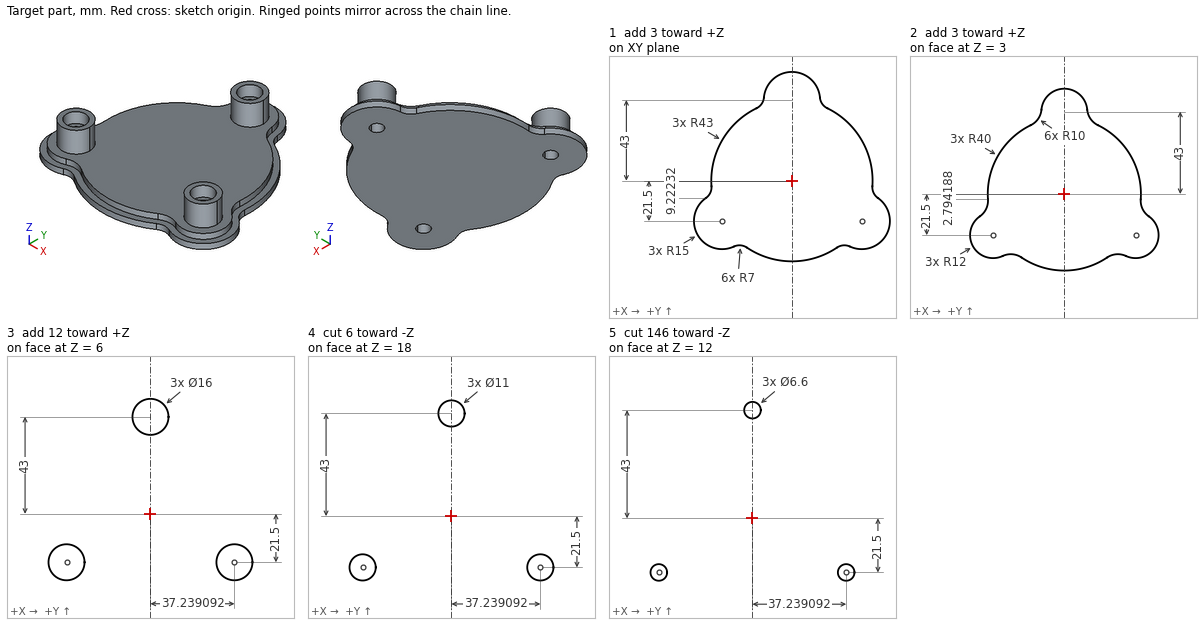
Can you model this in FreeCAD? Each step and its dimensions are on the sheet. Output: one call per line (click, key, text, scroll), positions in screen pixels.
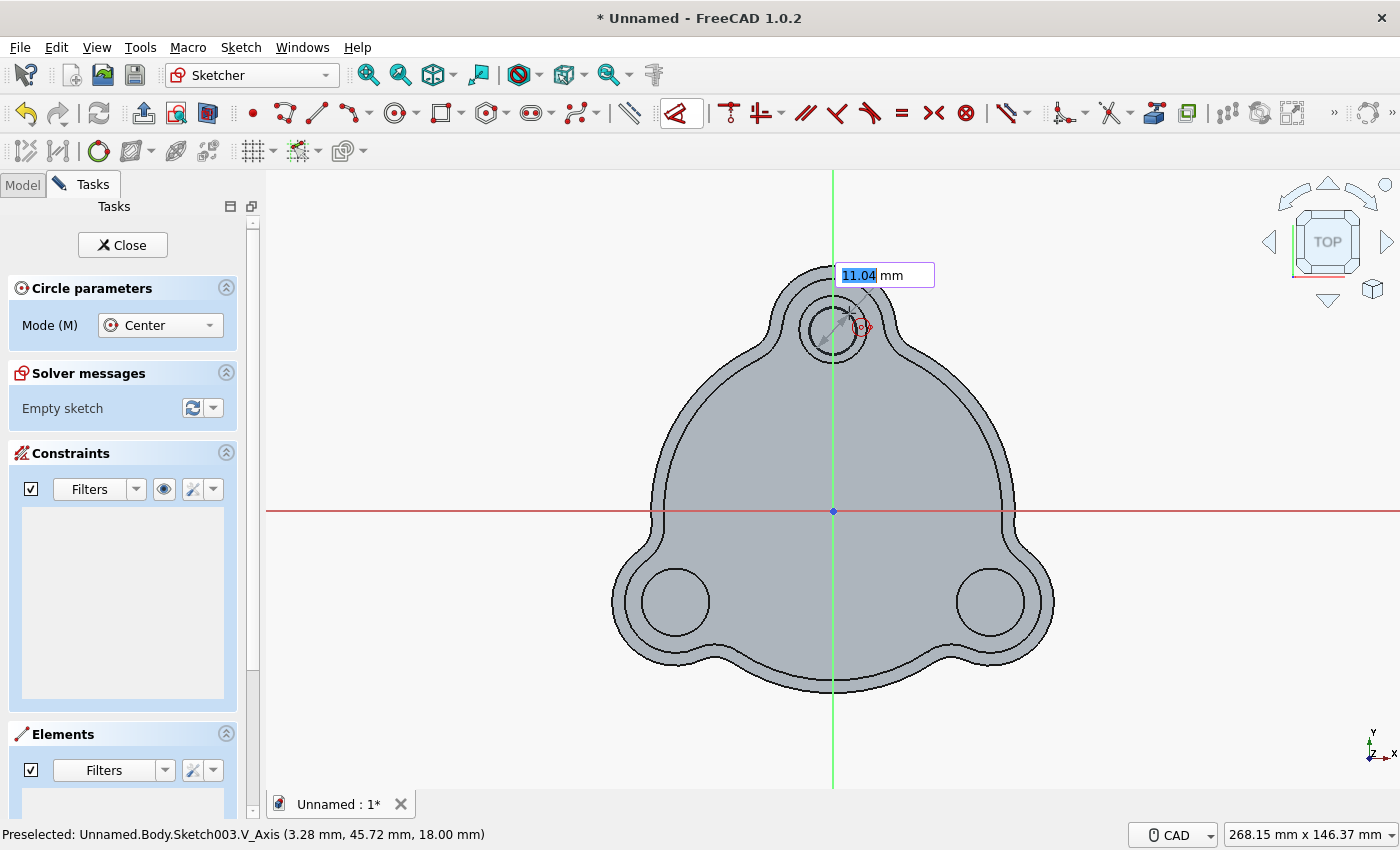
text(11)
key(Return)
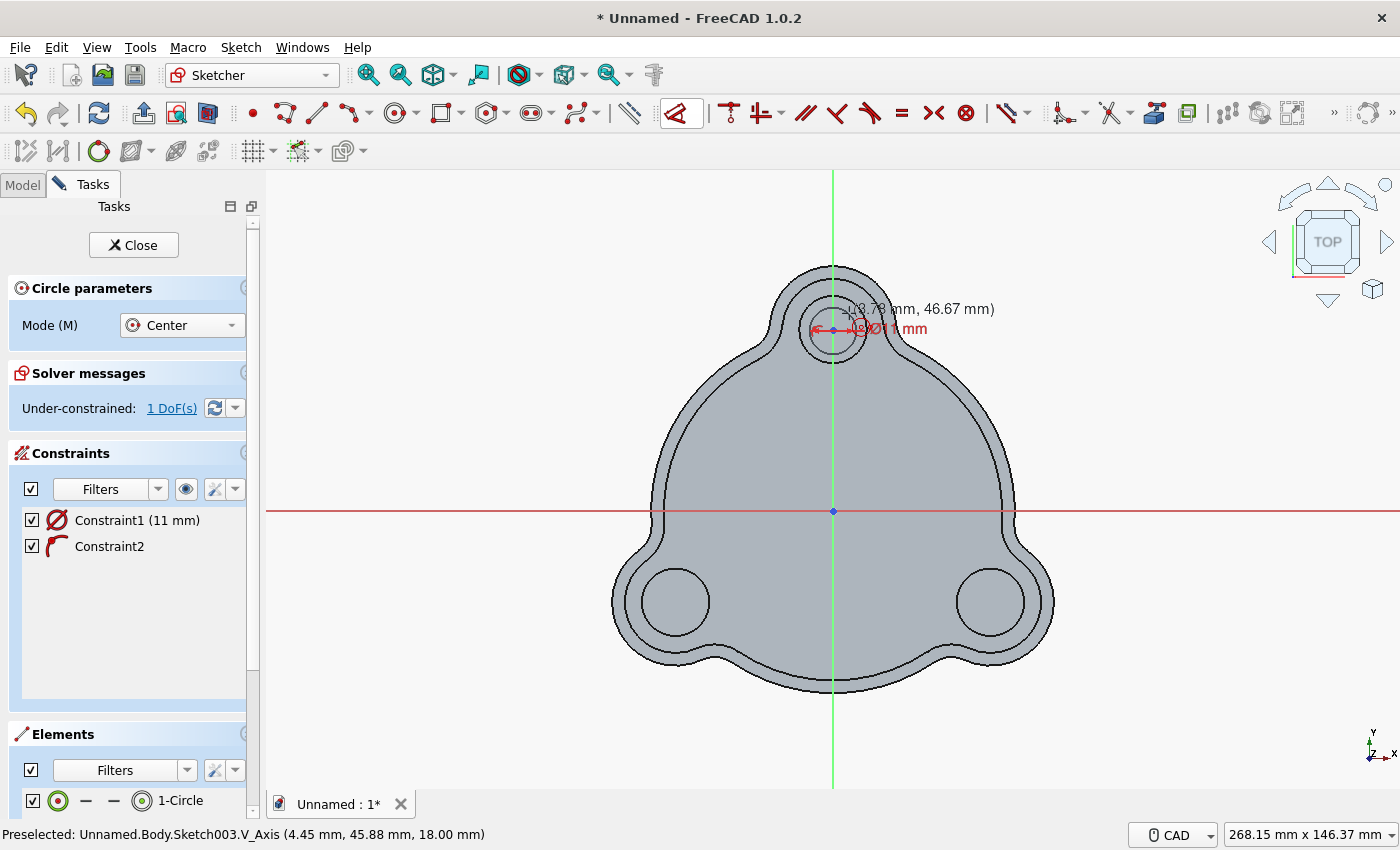
click(990, 602)
move(1007, 586)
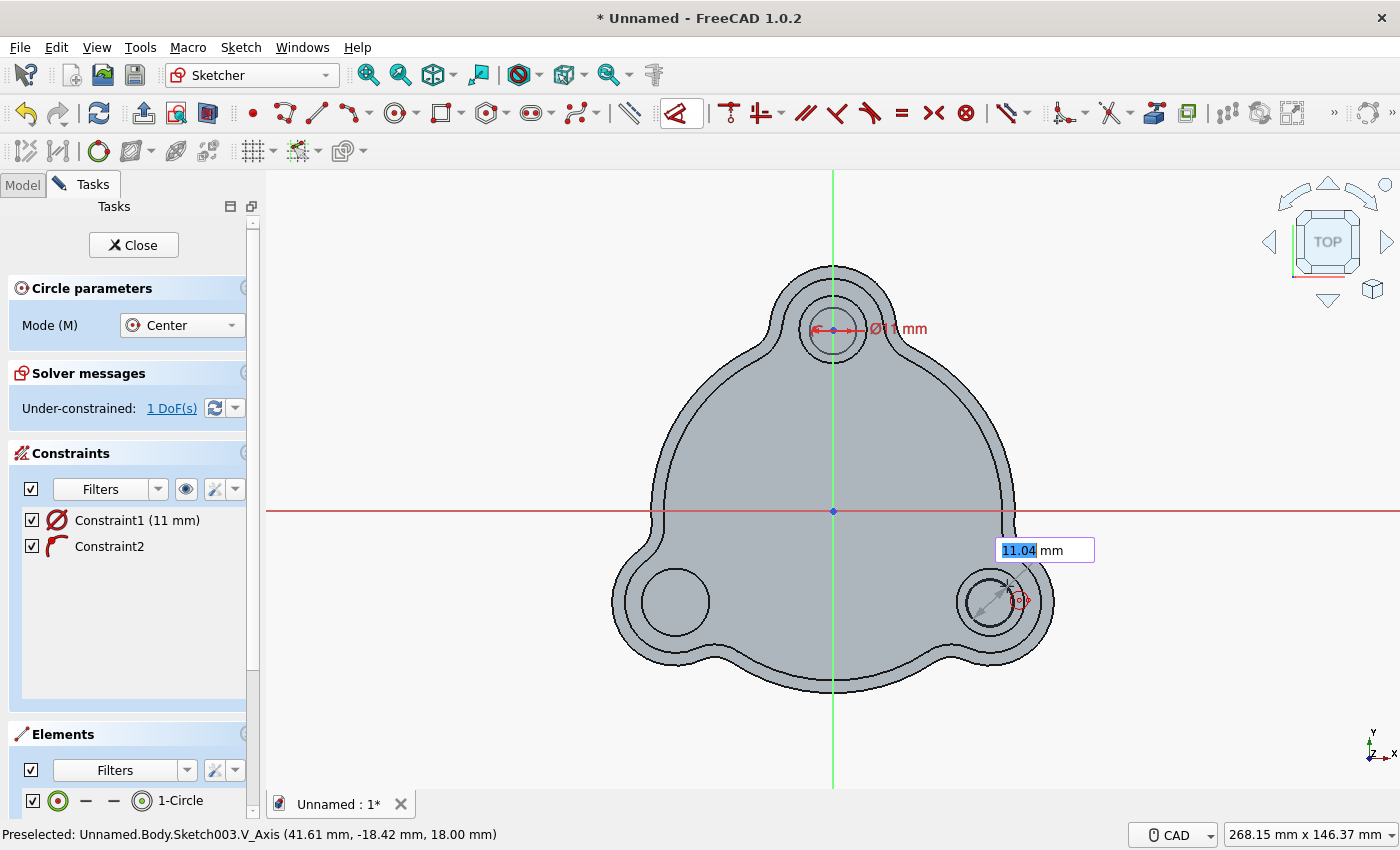
text(11)
key(Return)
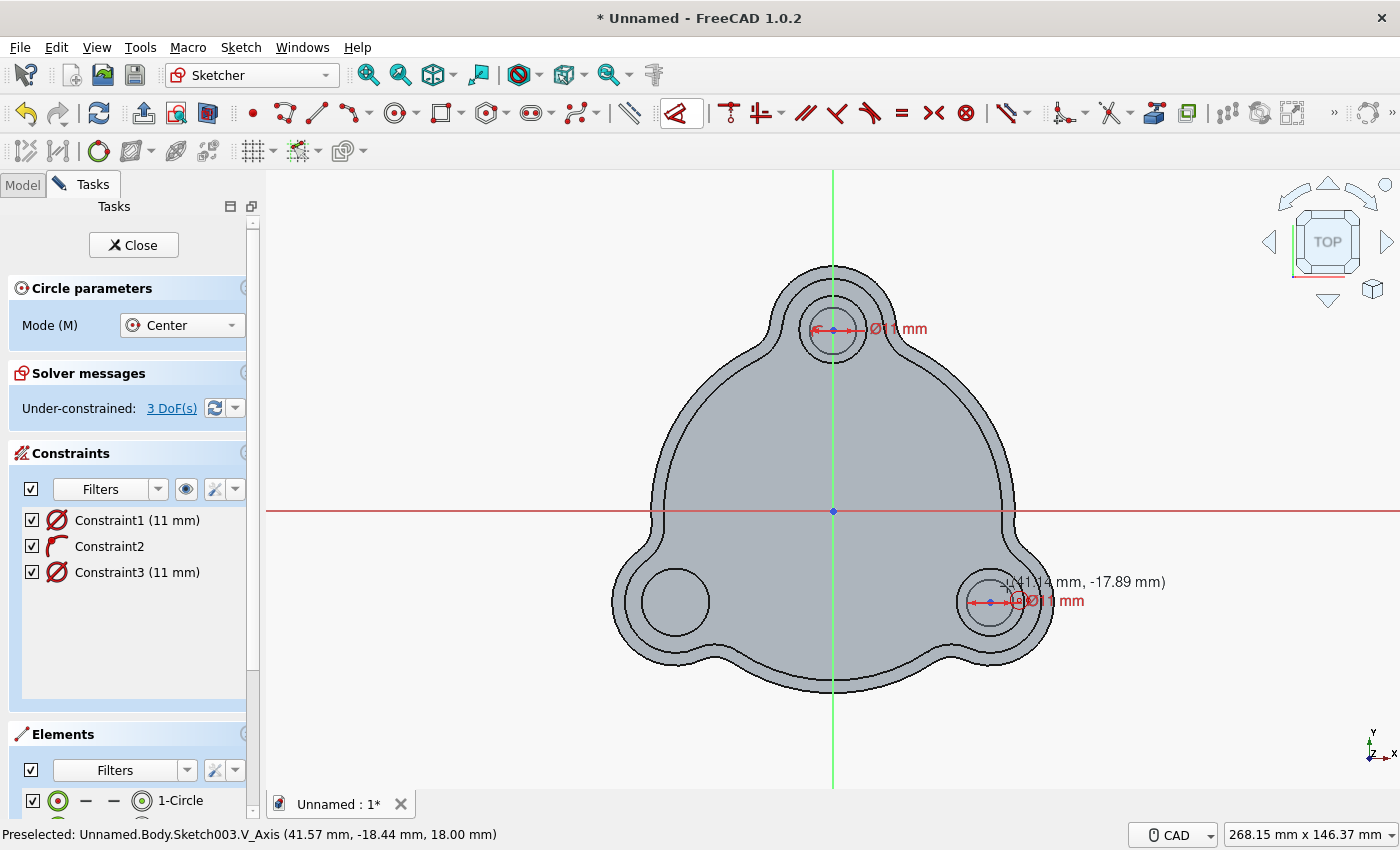
click(676, 602)
move(692, 586)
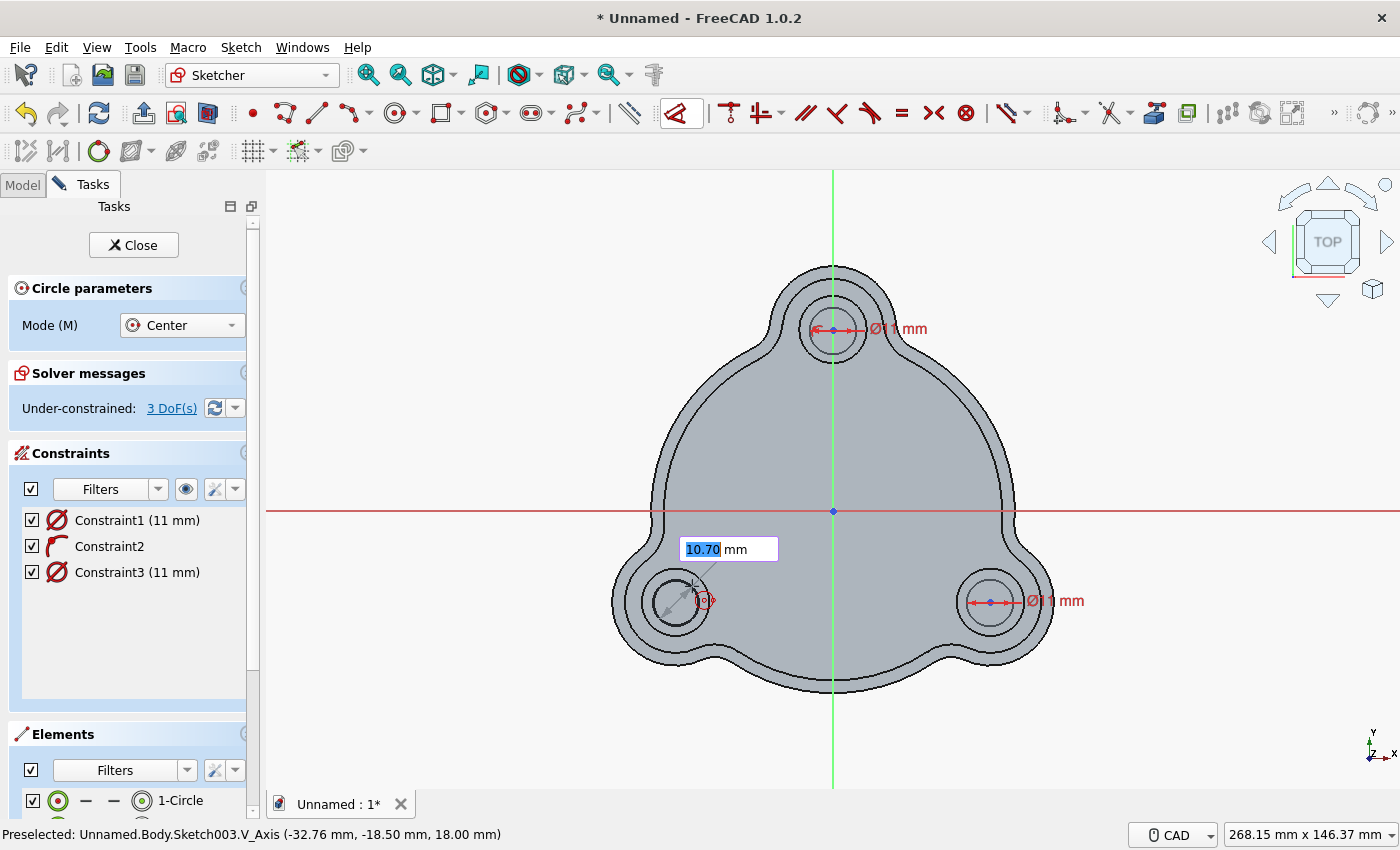
text(11)
key(Return)
key(Escape)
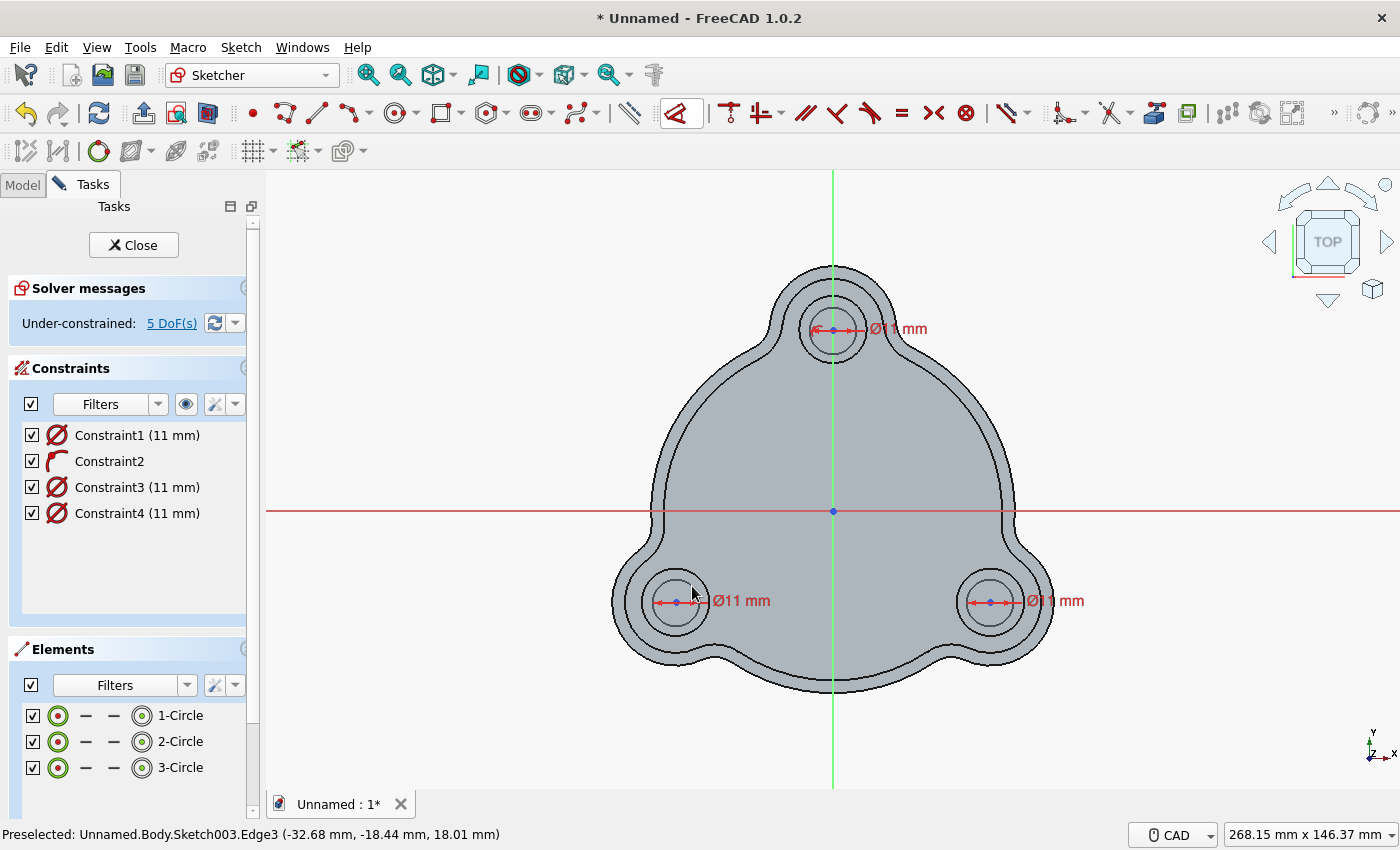
click(990, 603)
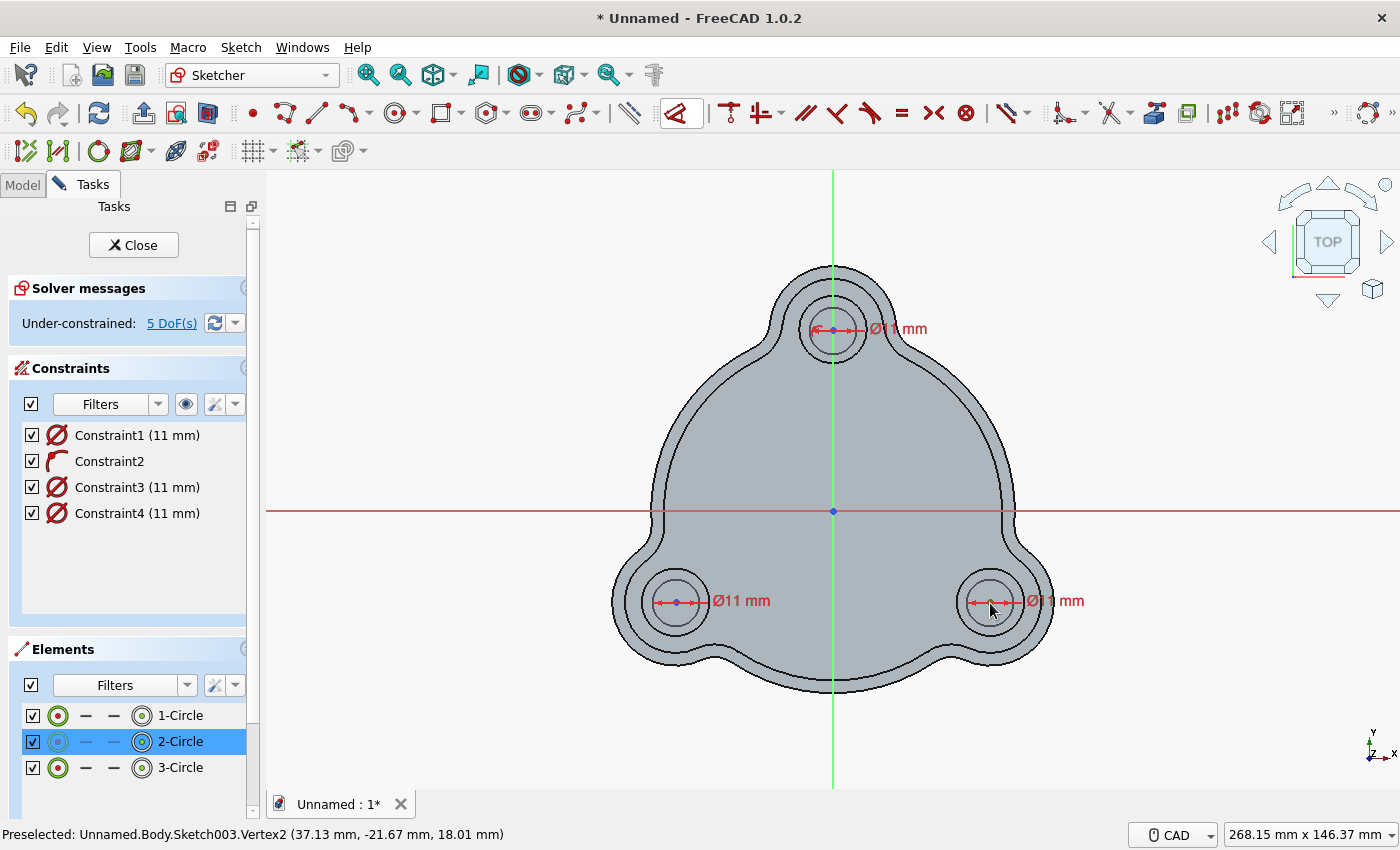
click(676, 603)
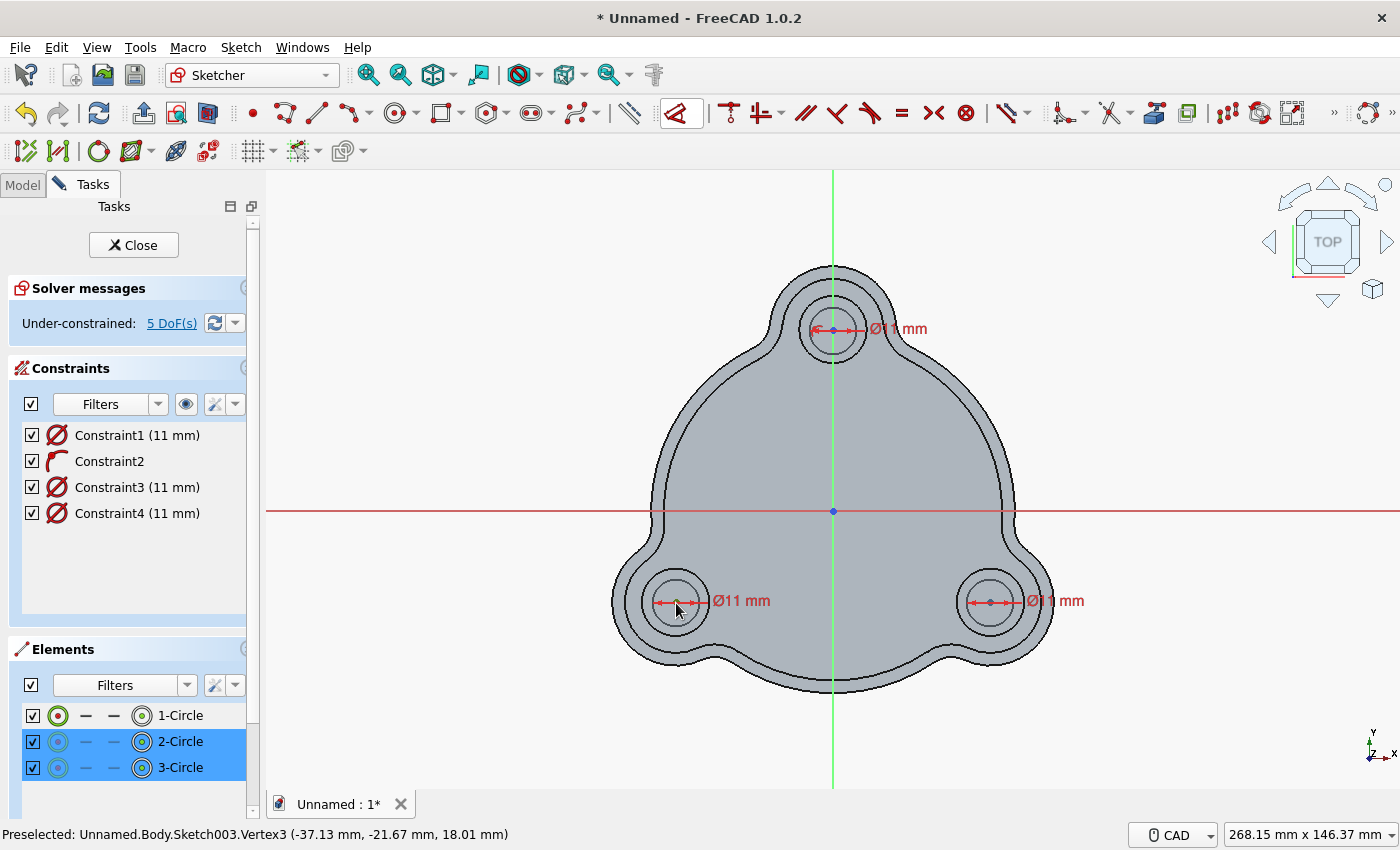
click(833, 721)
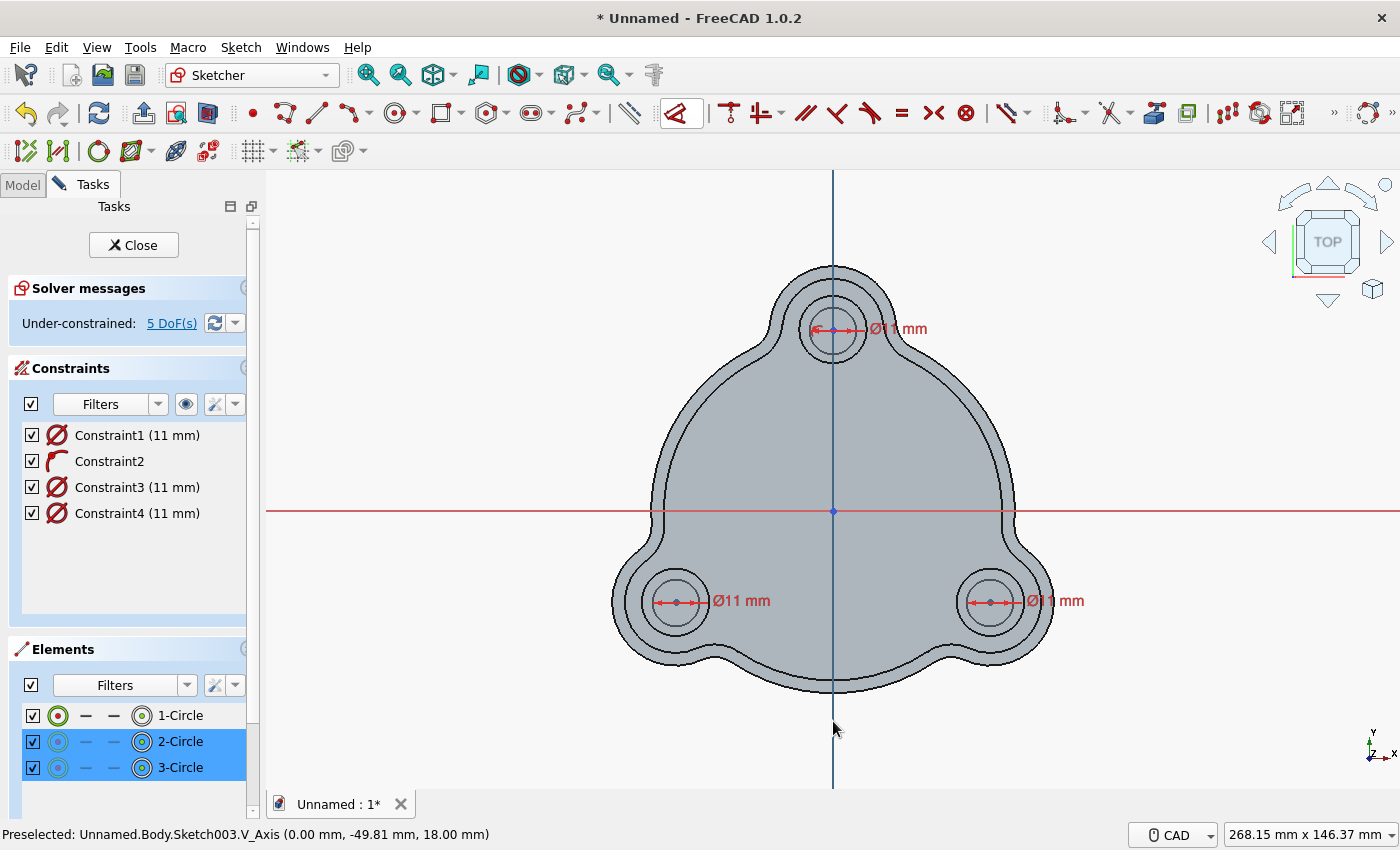
click(934, 114)